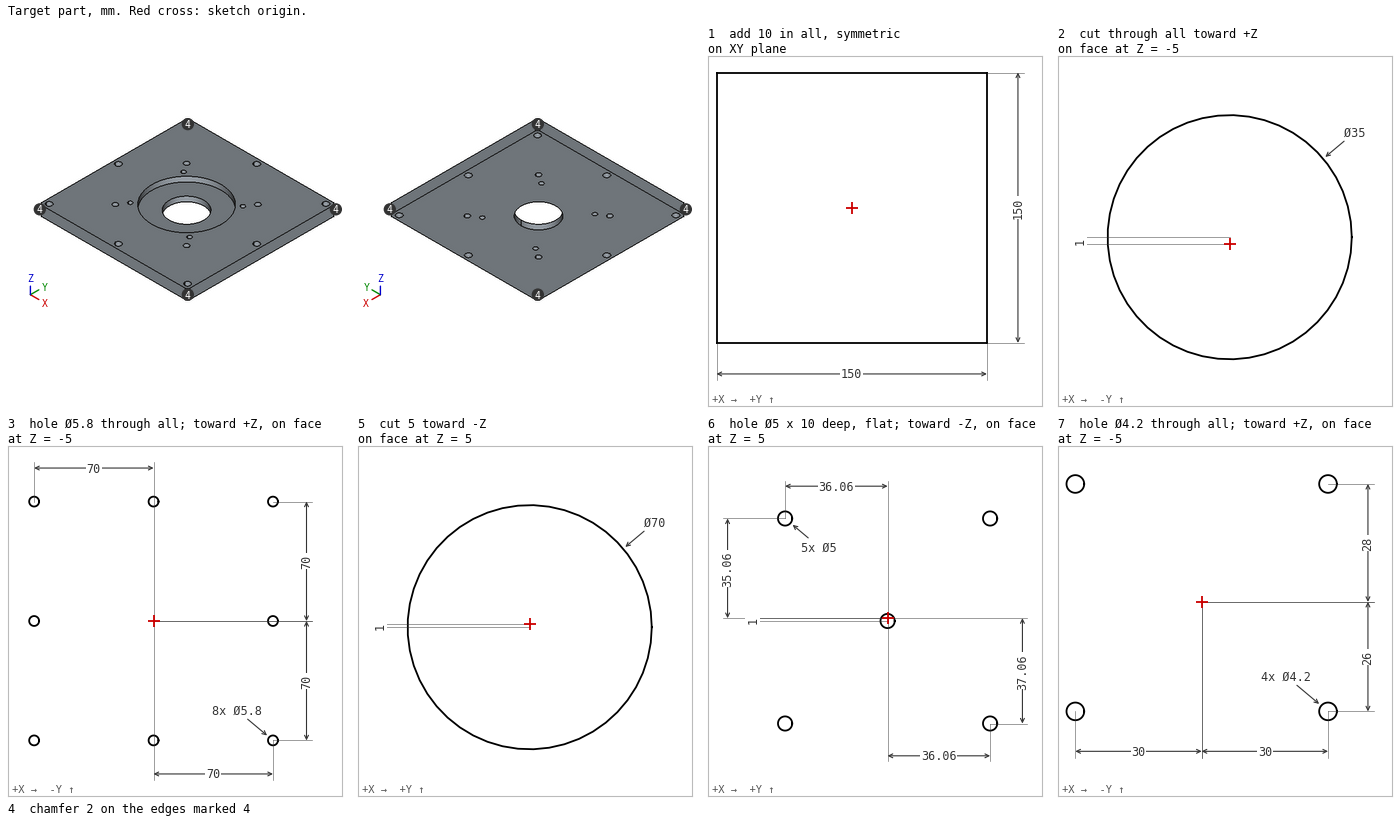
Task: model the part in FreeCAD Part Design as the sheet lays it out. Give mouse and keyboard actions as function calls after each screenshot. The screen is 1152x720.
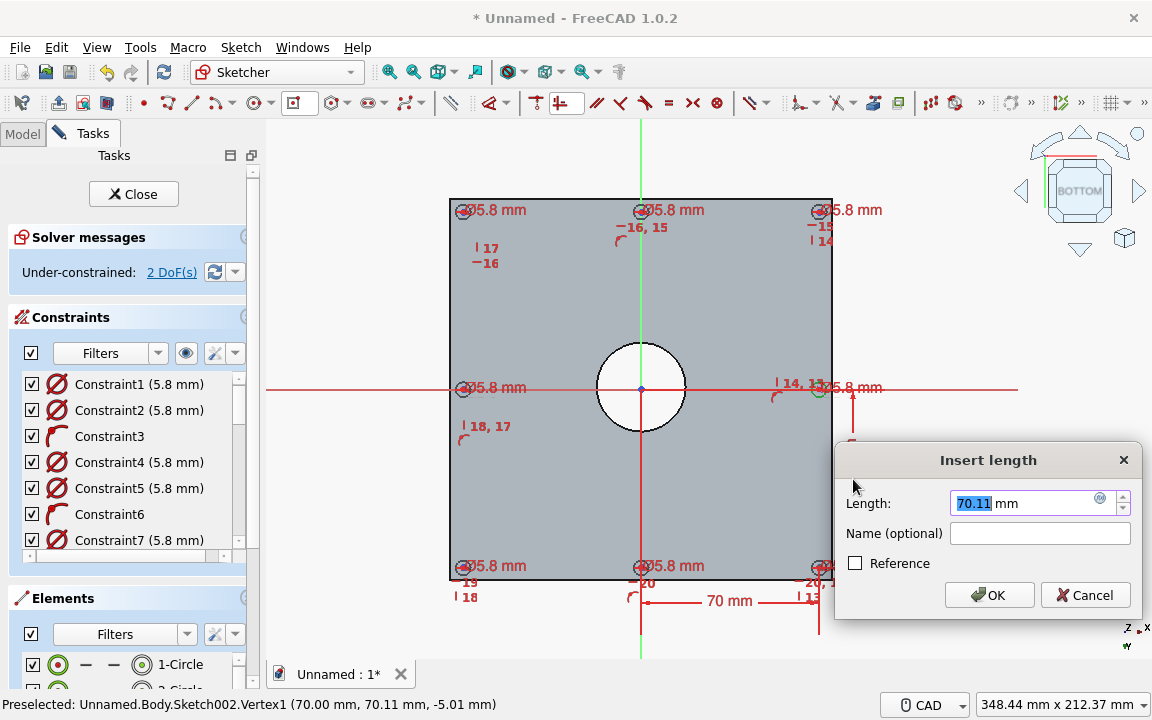
text(70)
key(Return)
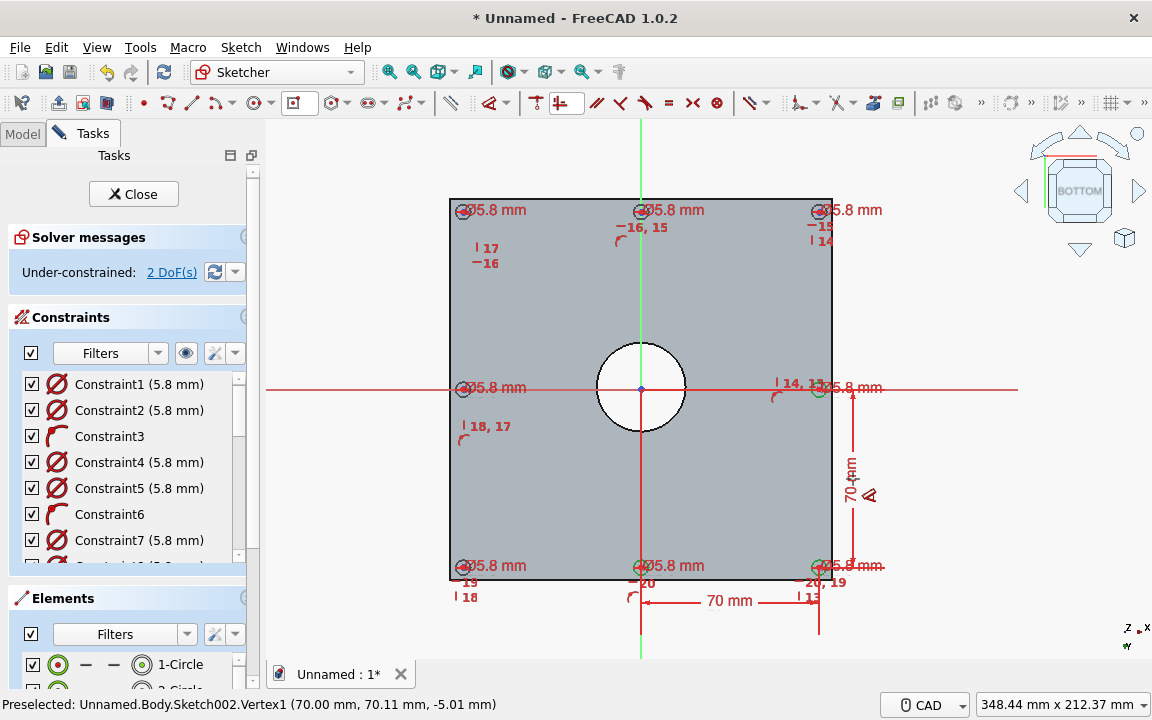
click(819, 212)
click(853, 301)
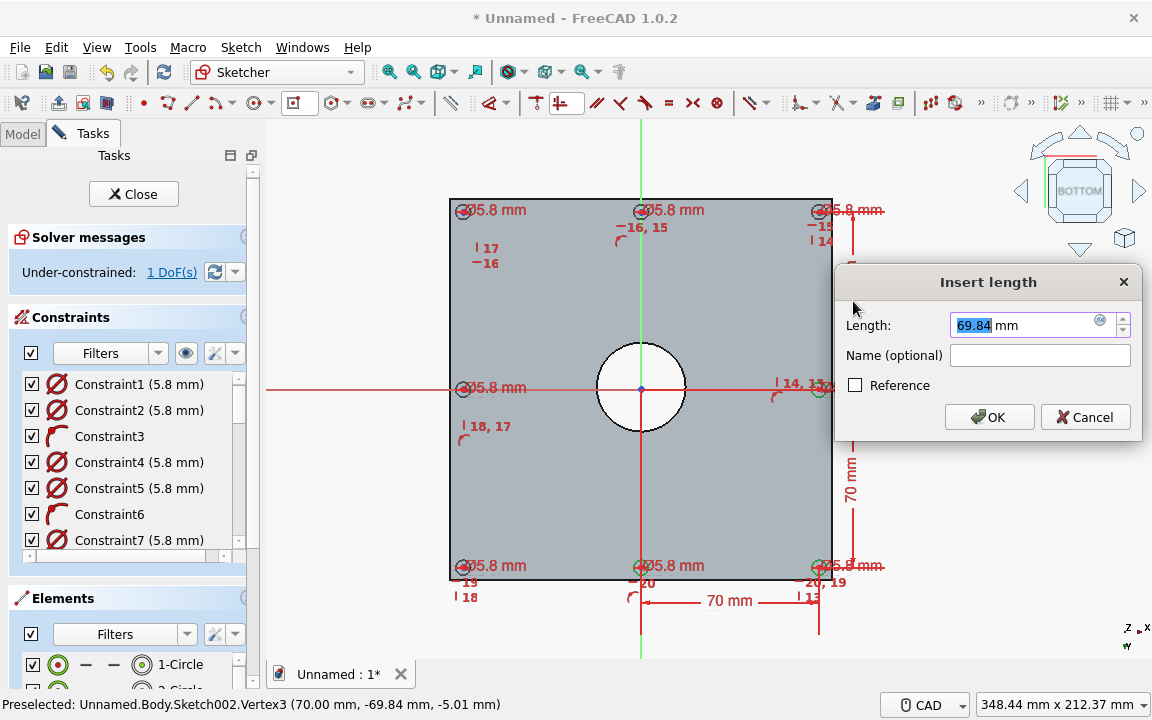
text(70)
key(Return)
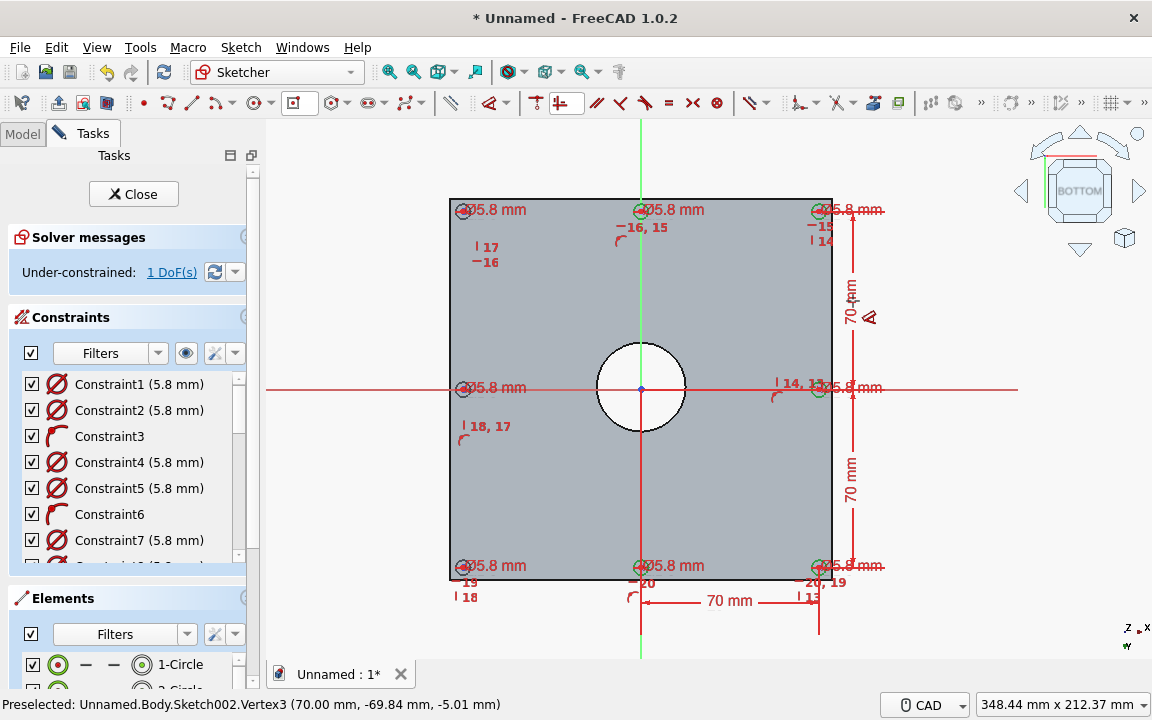
click(463, 212)
click(552, 178)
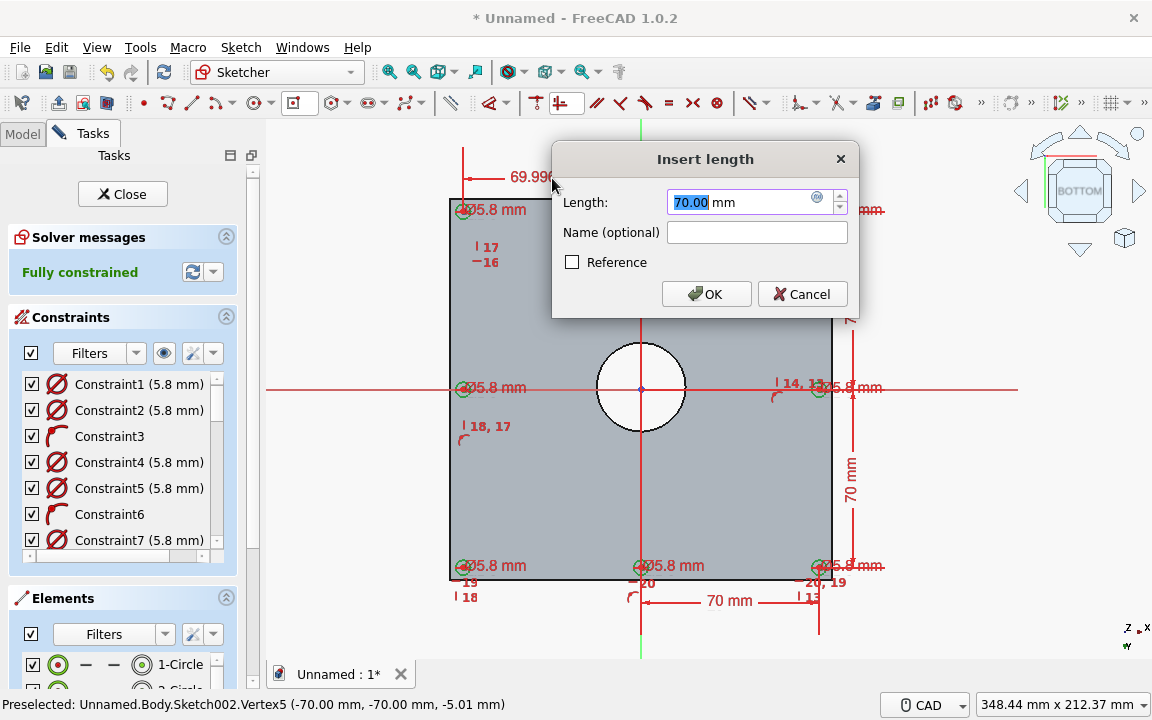
text(70)
key(Return)
key(Escape)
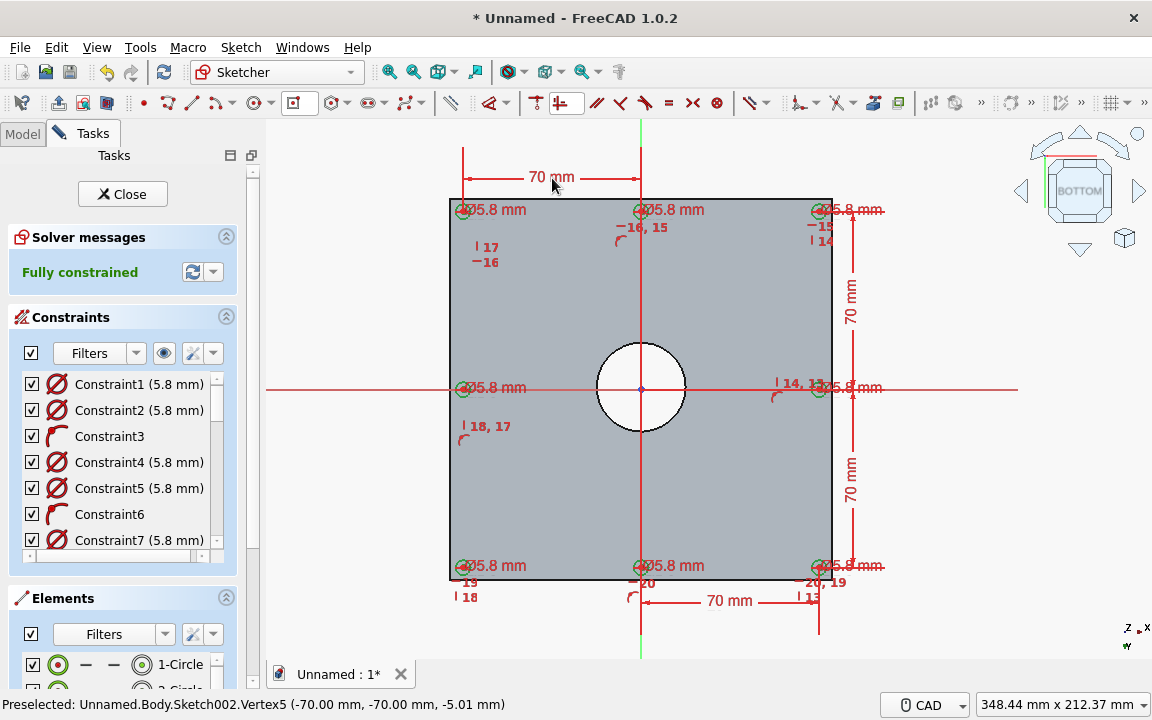
click(123, 194)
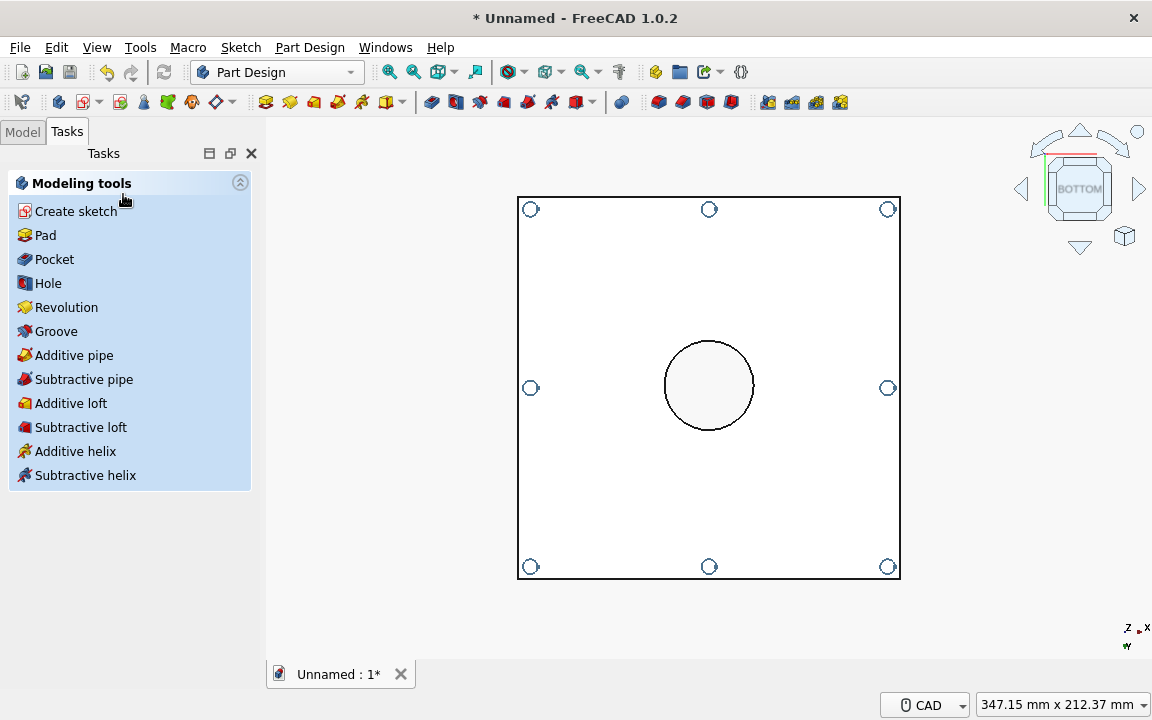
click(456, 102)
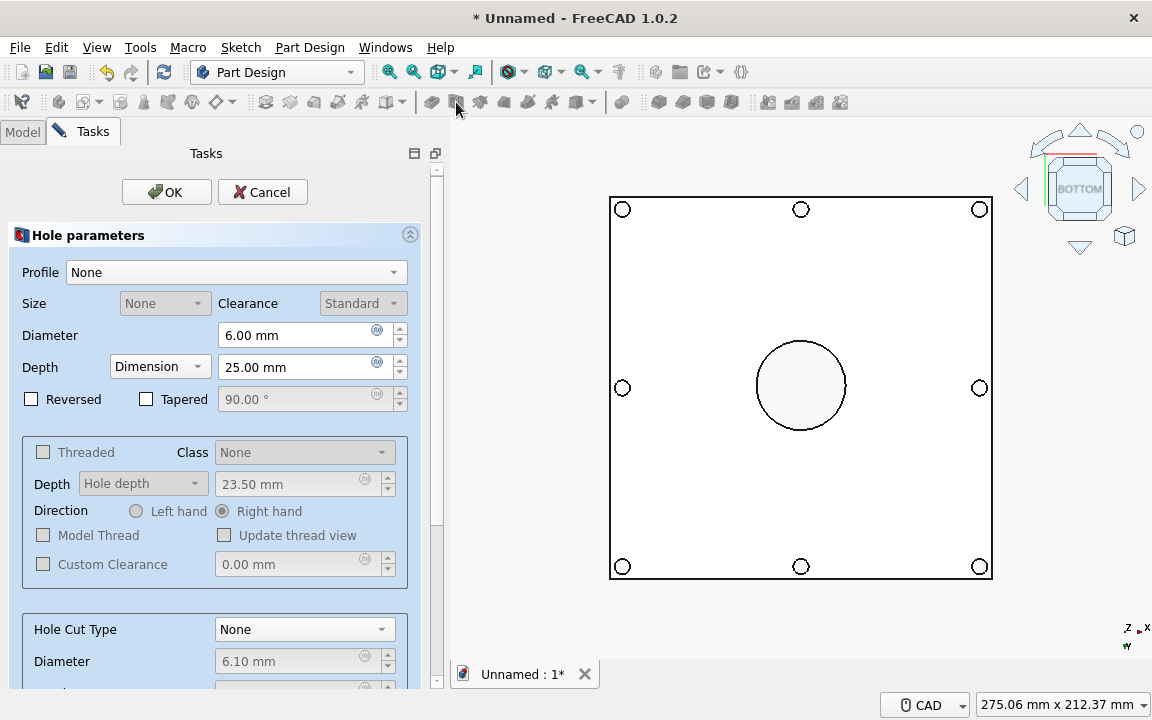
triple_click(305, 335)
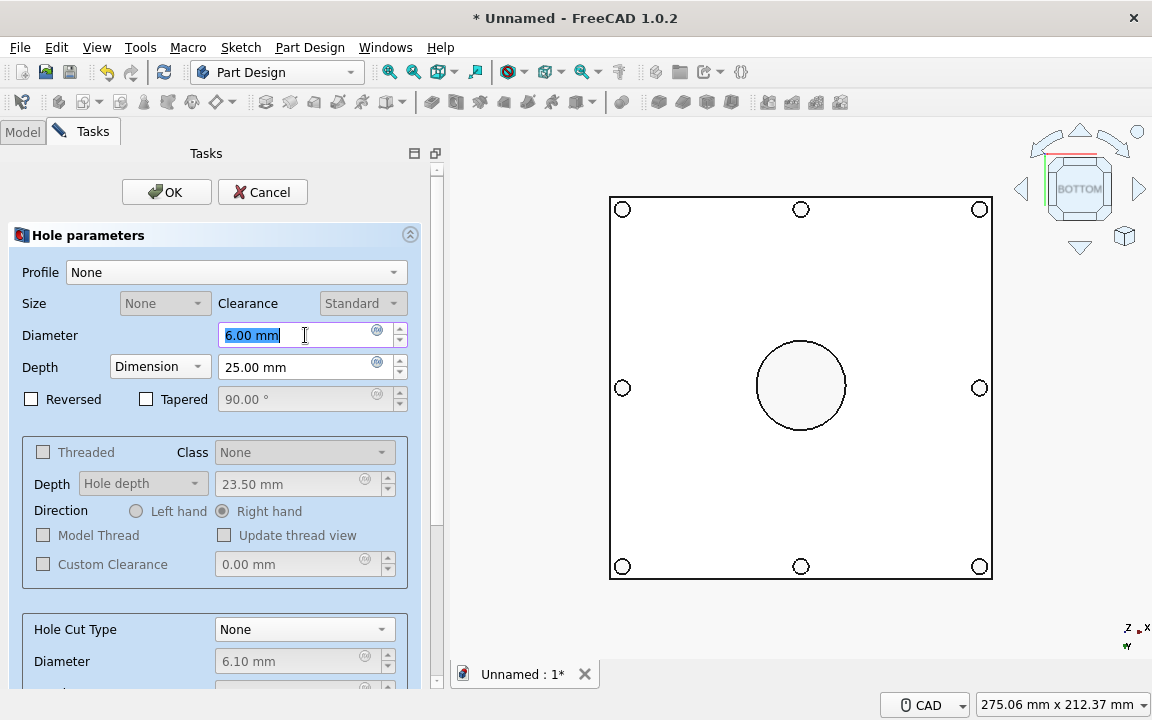
text(5.8)
key(Tab)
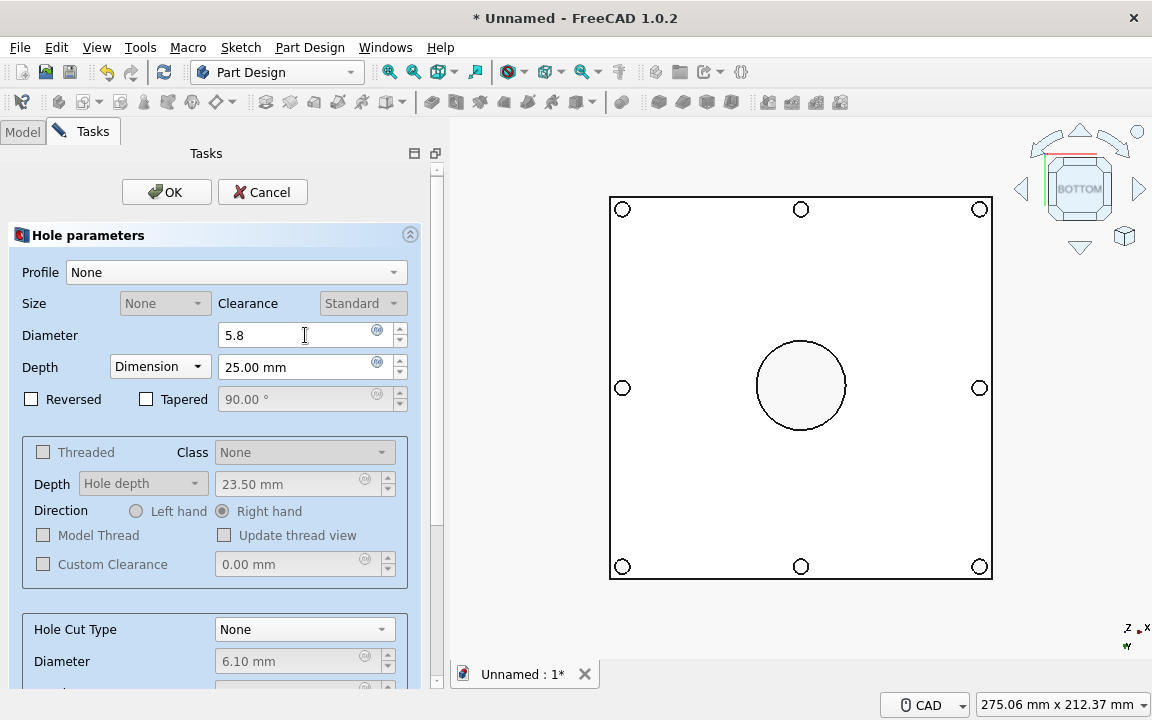
click(161, 366)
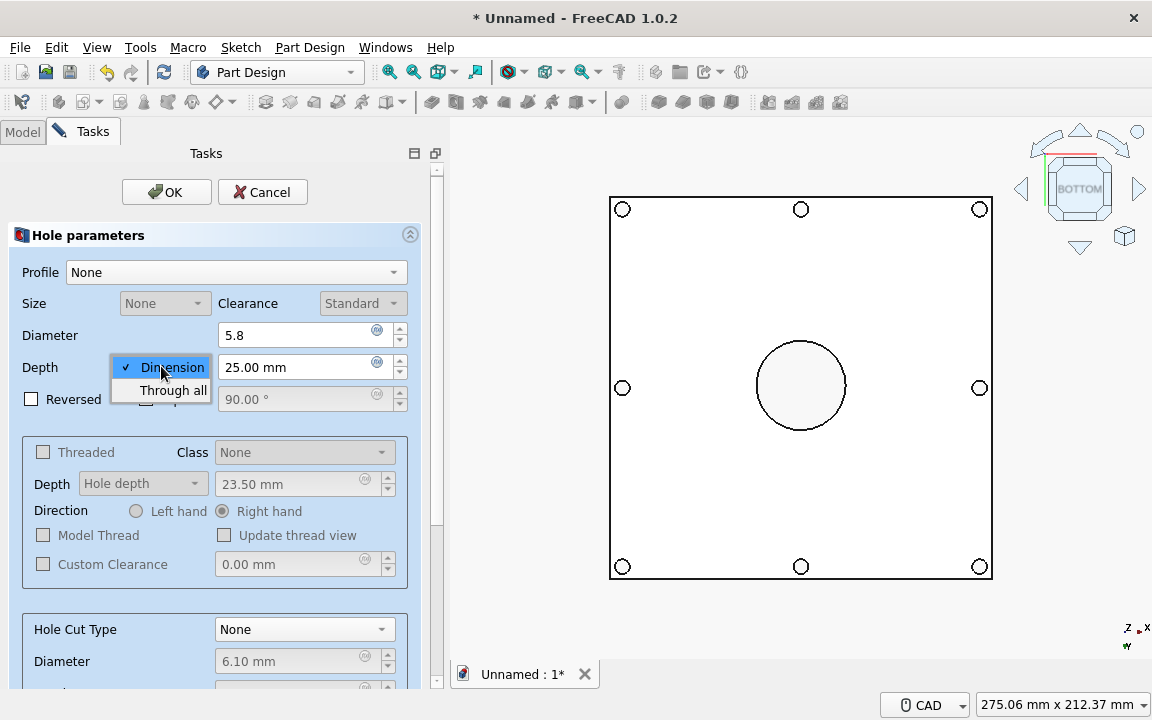
click(160, 390)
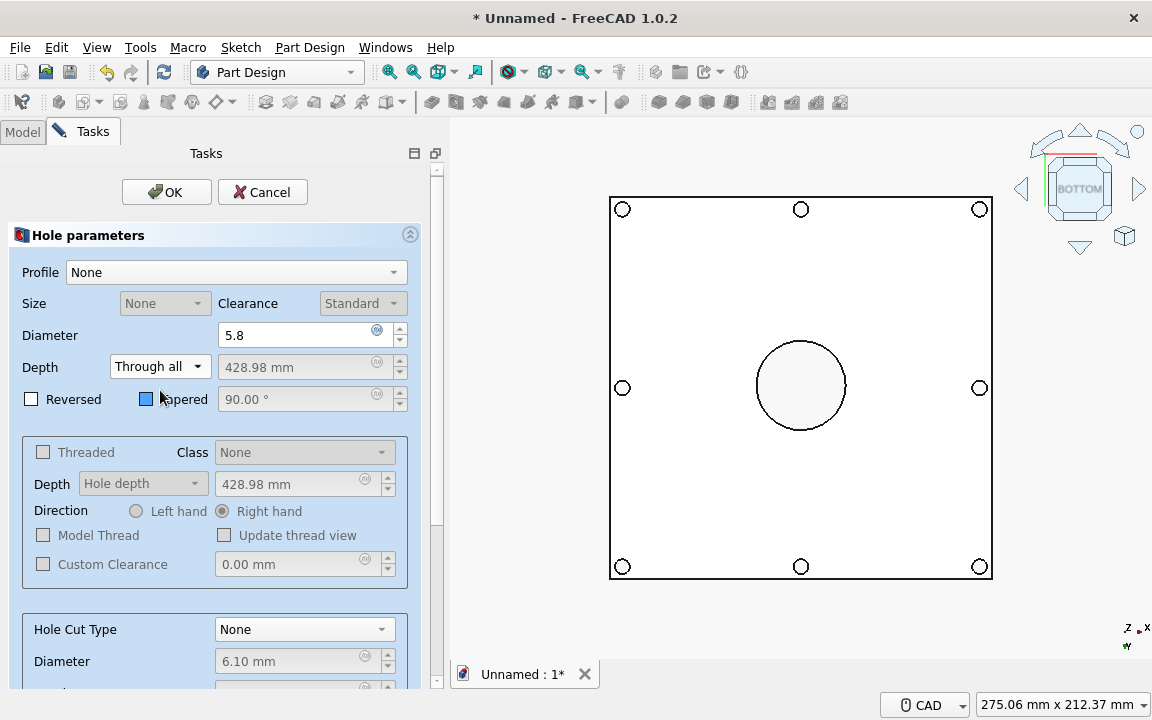
click(167, 192)